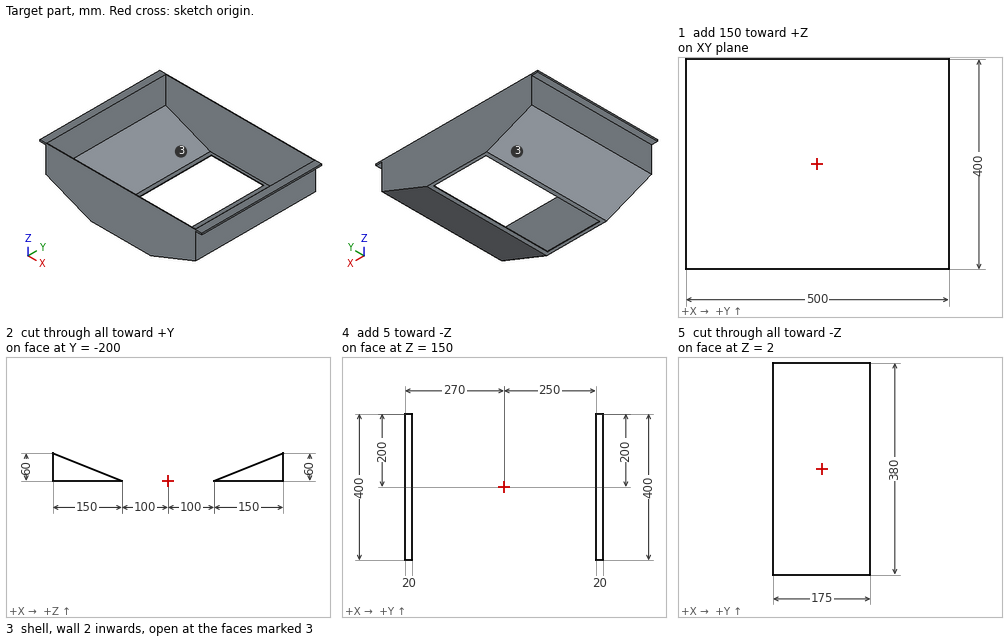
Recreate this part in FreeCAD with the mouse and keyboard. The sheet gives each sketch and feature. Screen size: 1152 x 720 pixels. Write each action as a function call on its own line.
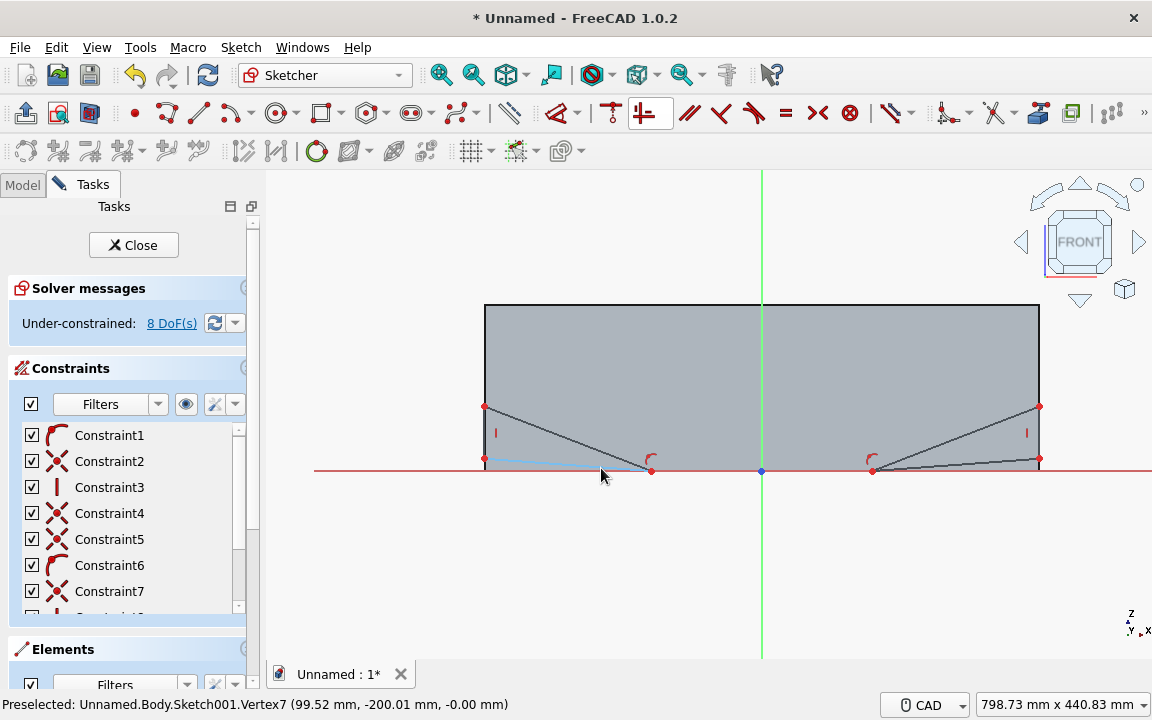
click(601, 467)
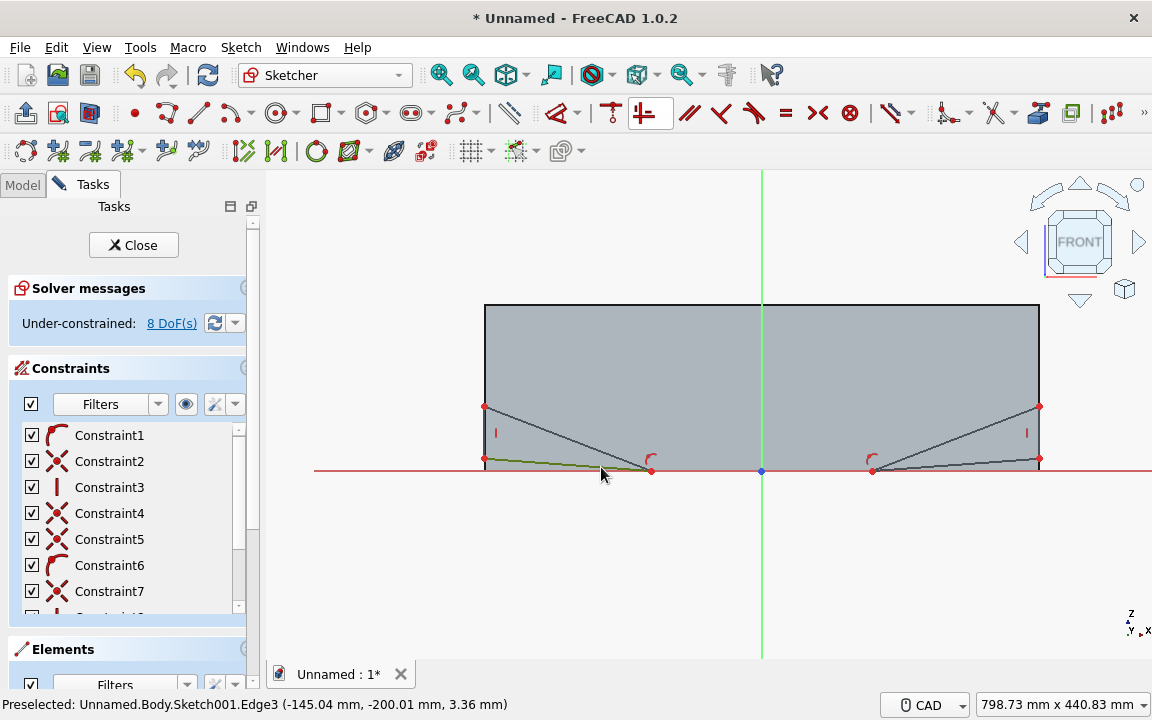
key(h)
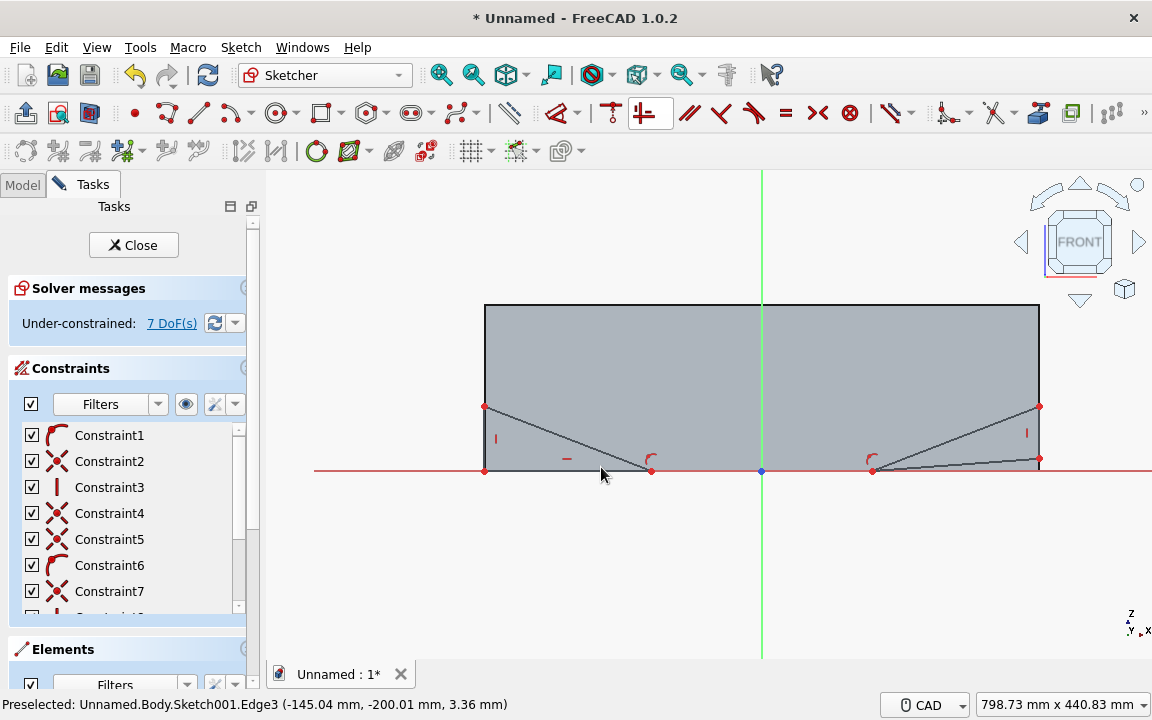
click(922, 467)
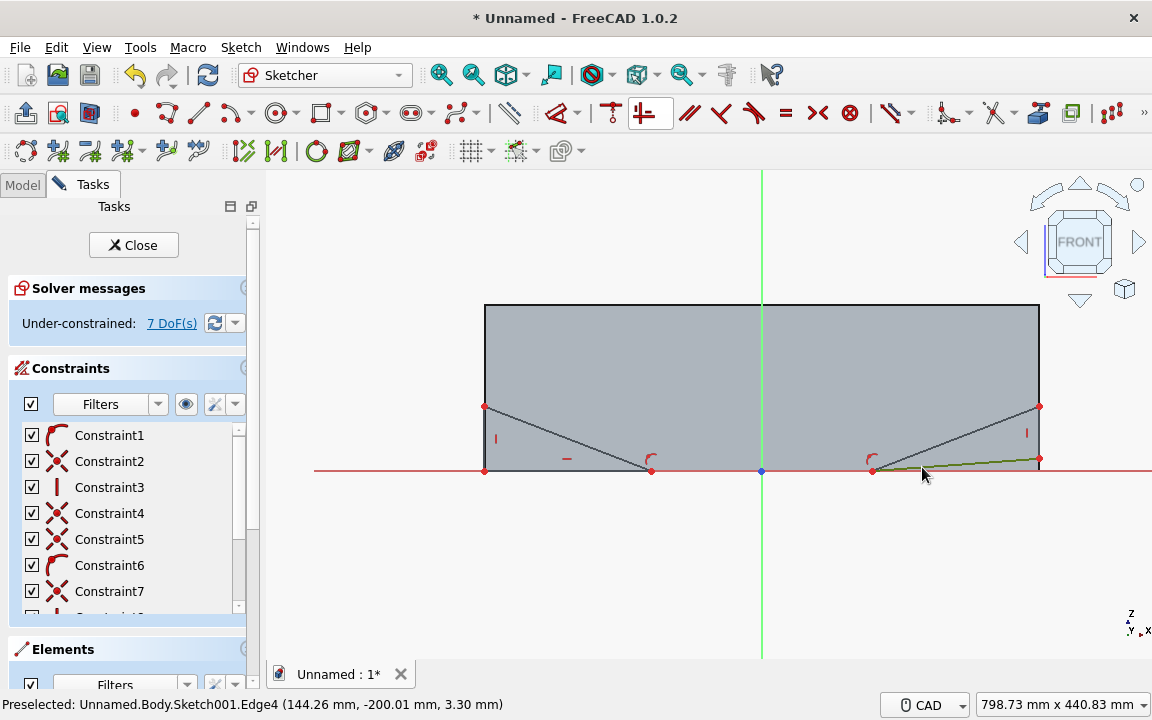
key(h)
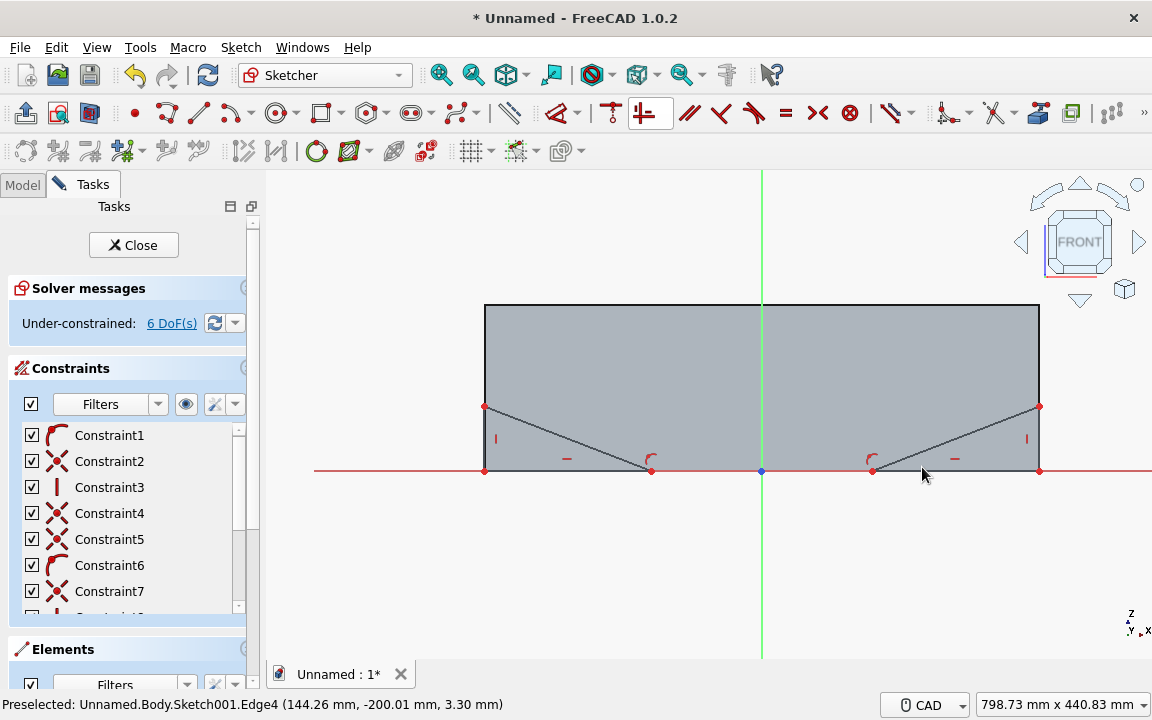
click(484, 426)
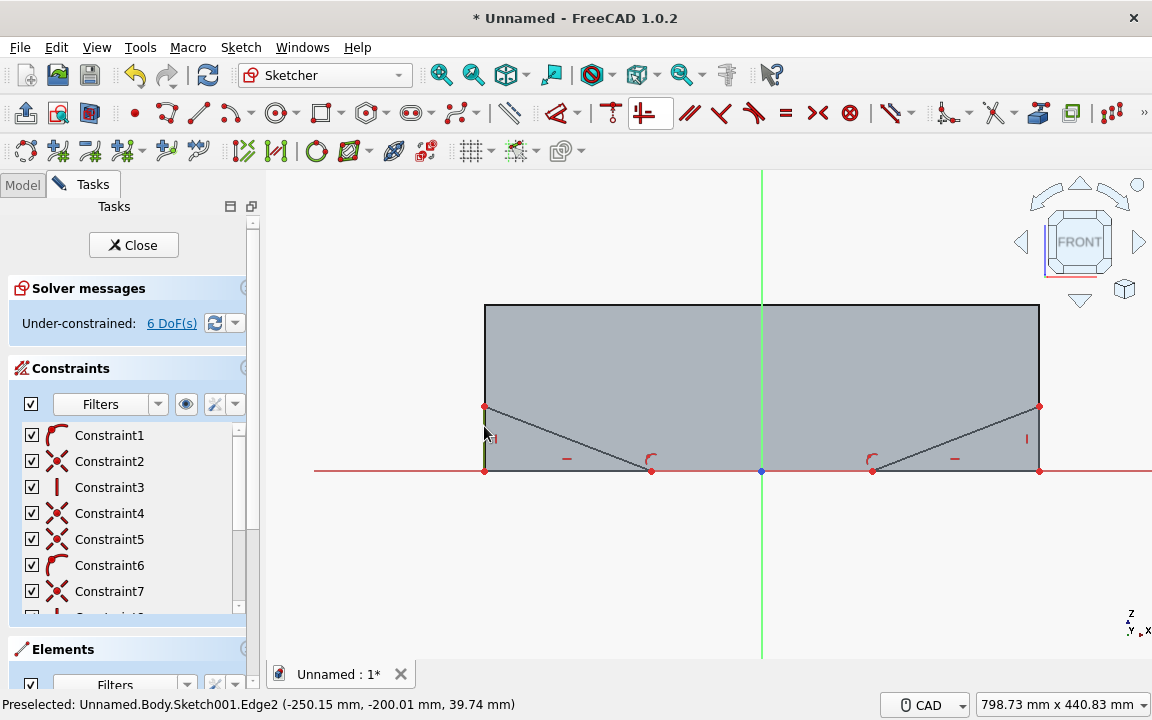
key(i)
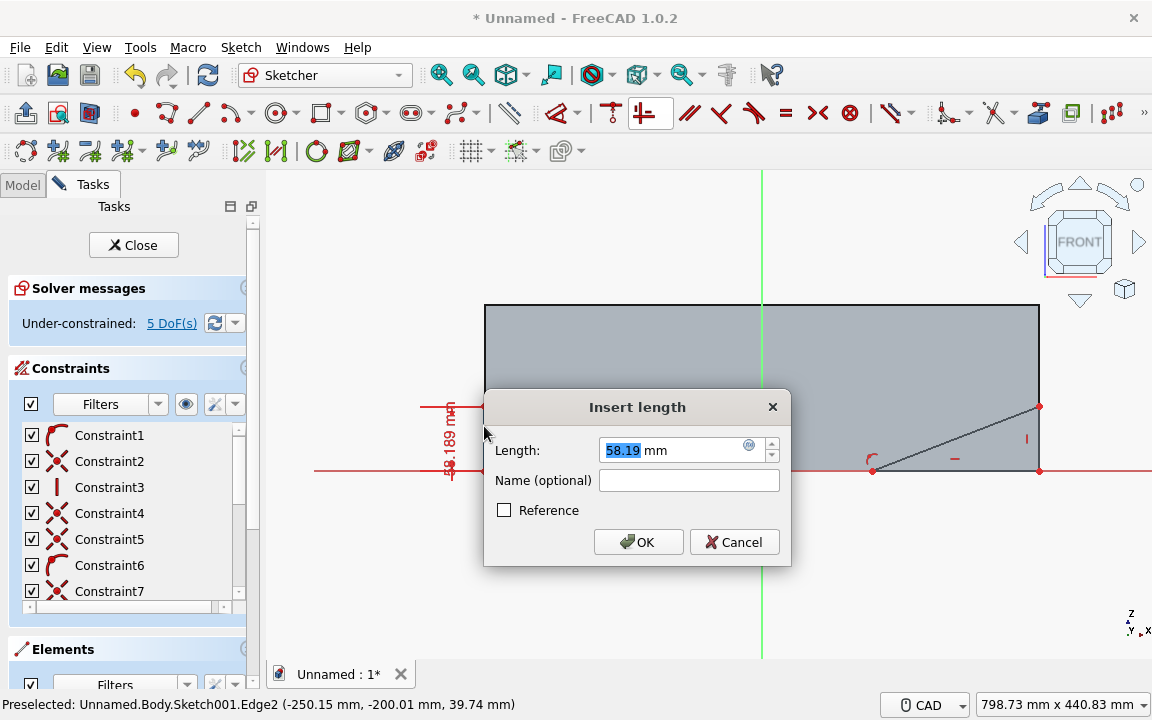
text(60)
key(Return)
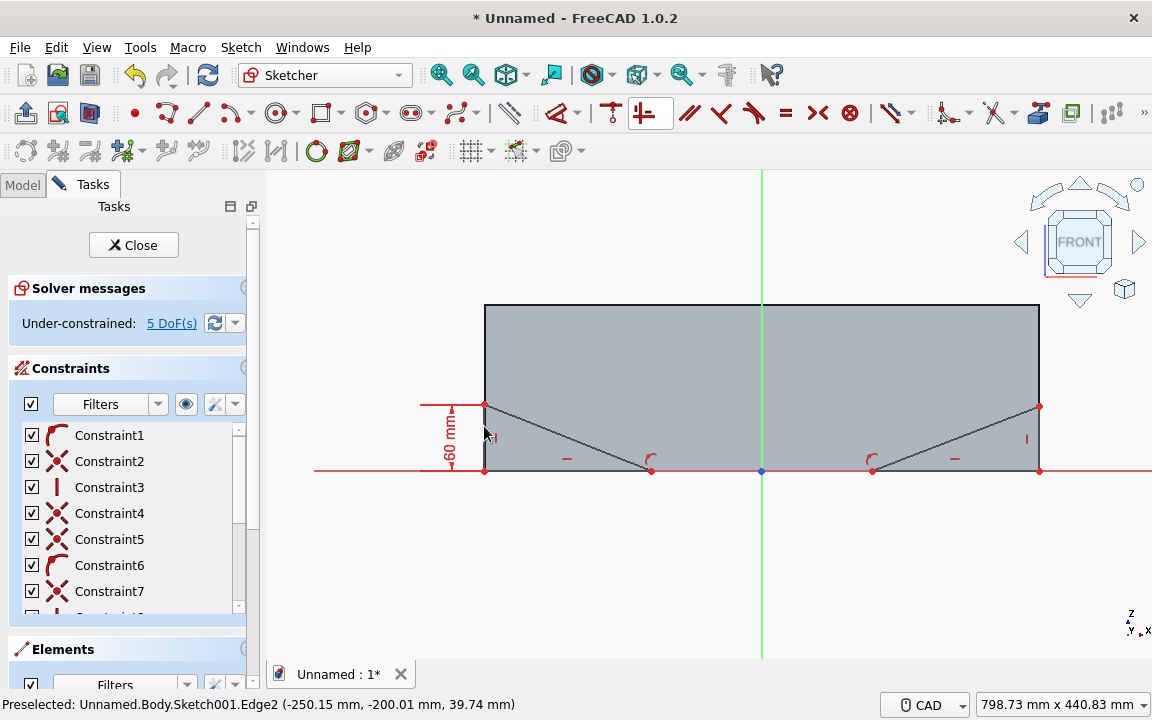
scroll(294, 309, down, 1)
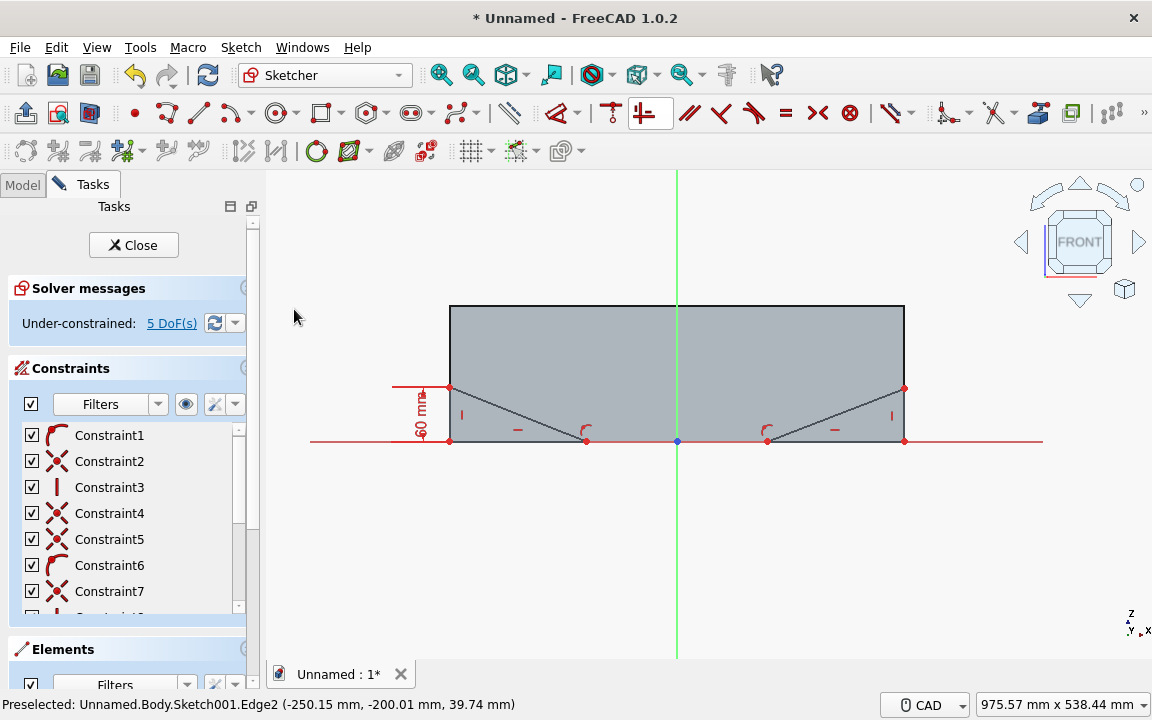
click(904, 426)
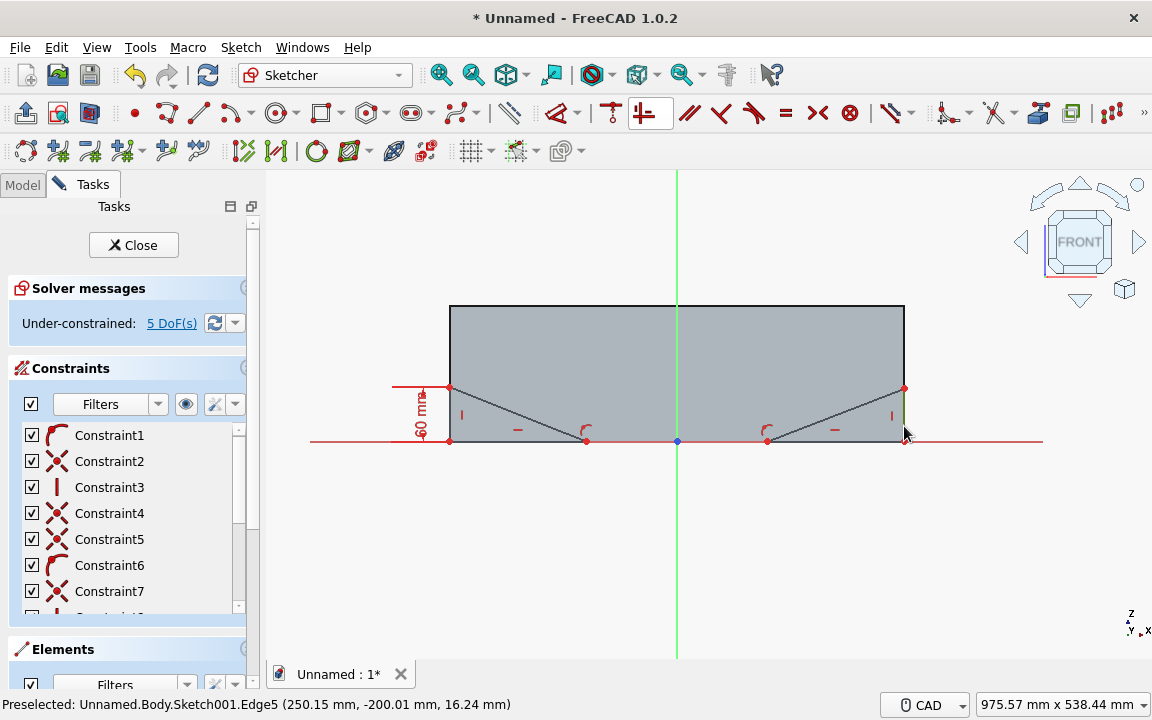
click(580, 114)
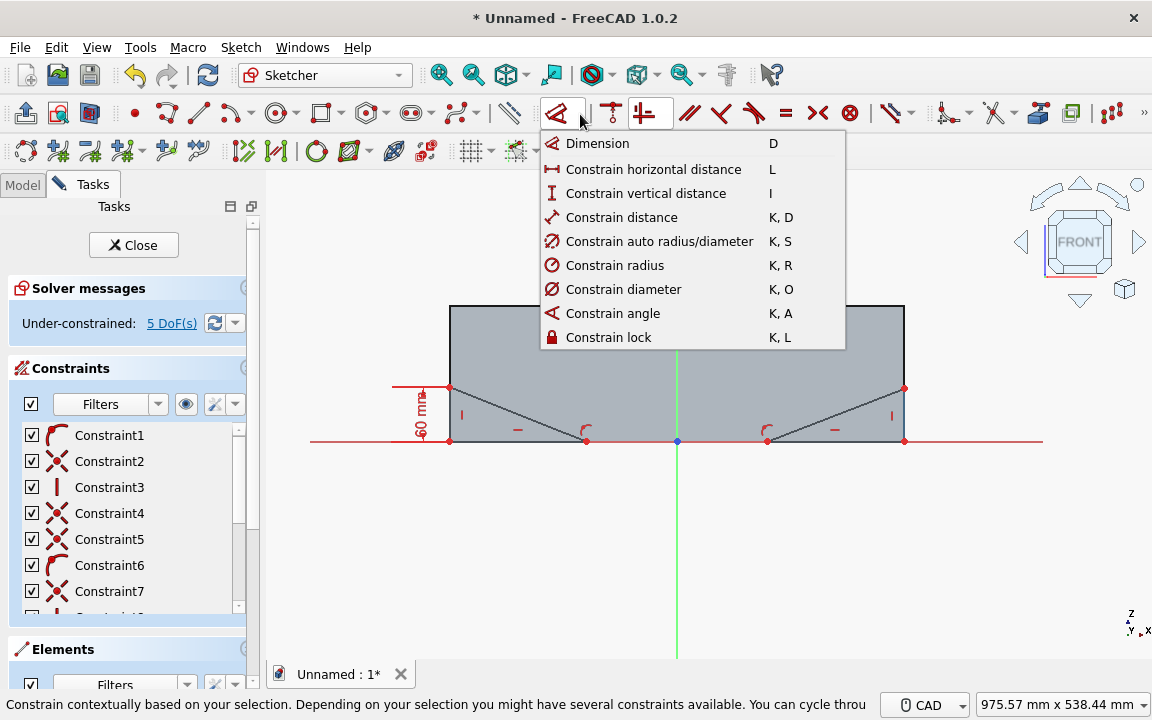
click(693, 193)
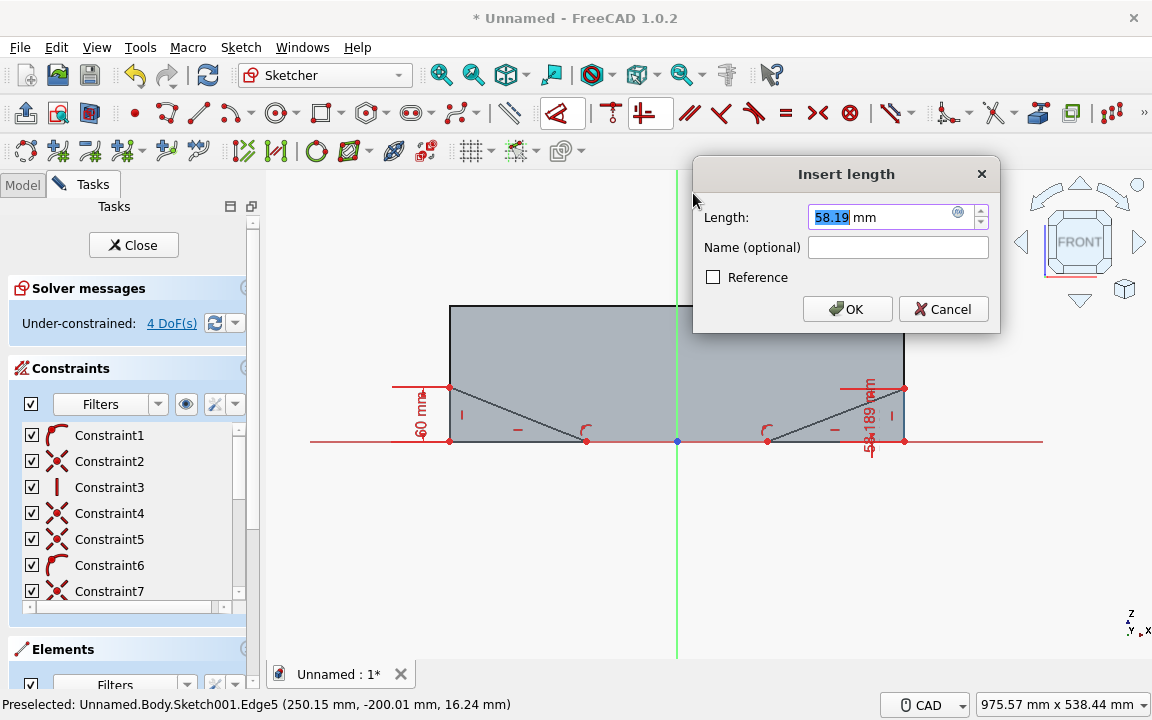
text(60)
key(Return)